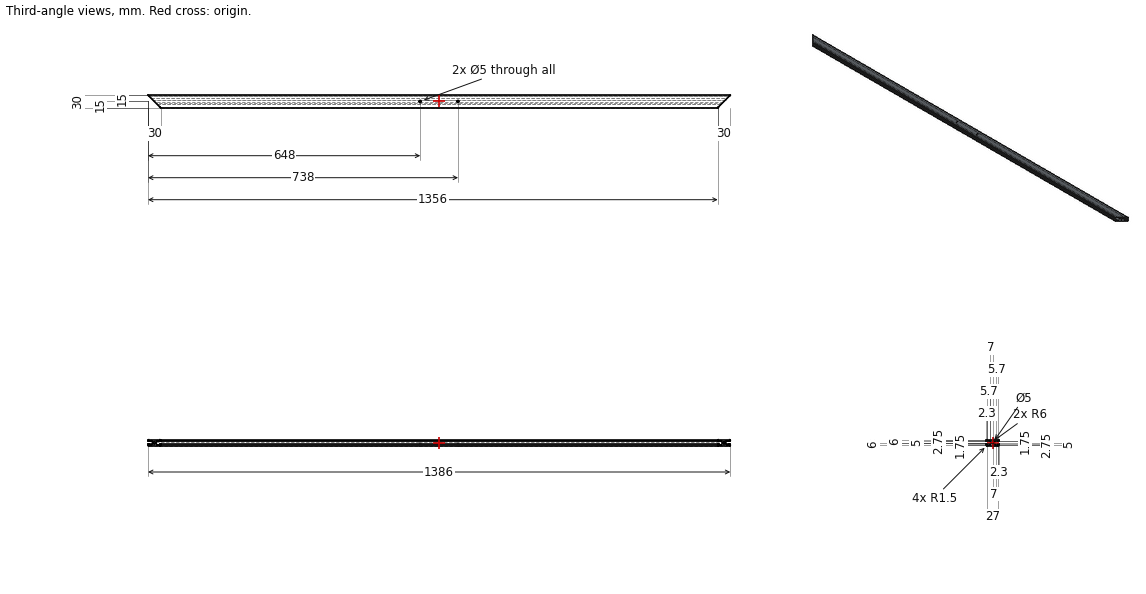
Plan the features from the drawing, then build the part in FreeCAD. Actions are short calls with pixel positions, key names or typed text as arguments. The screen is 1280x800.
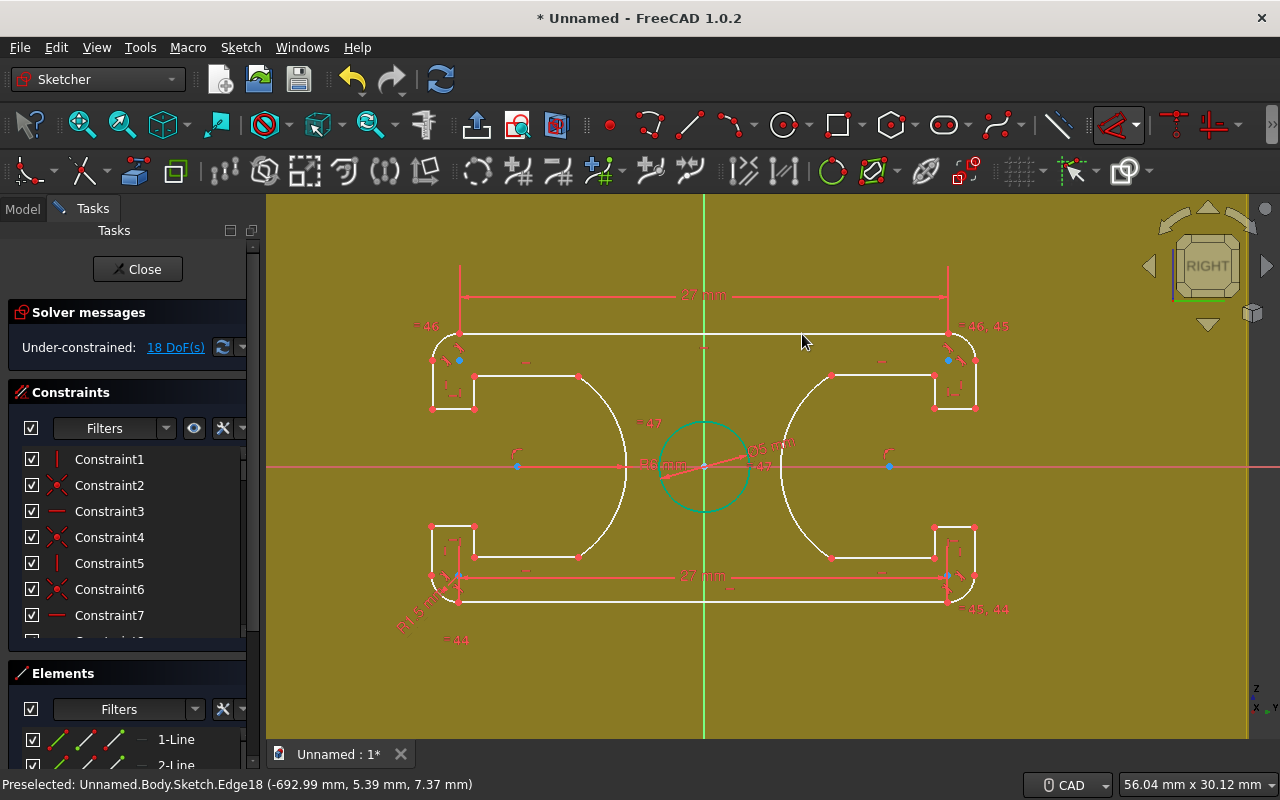
click(433, 361)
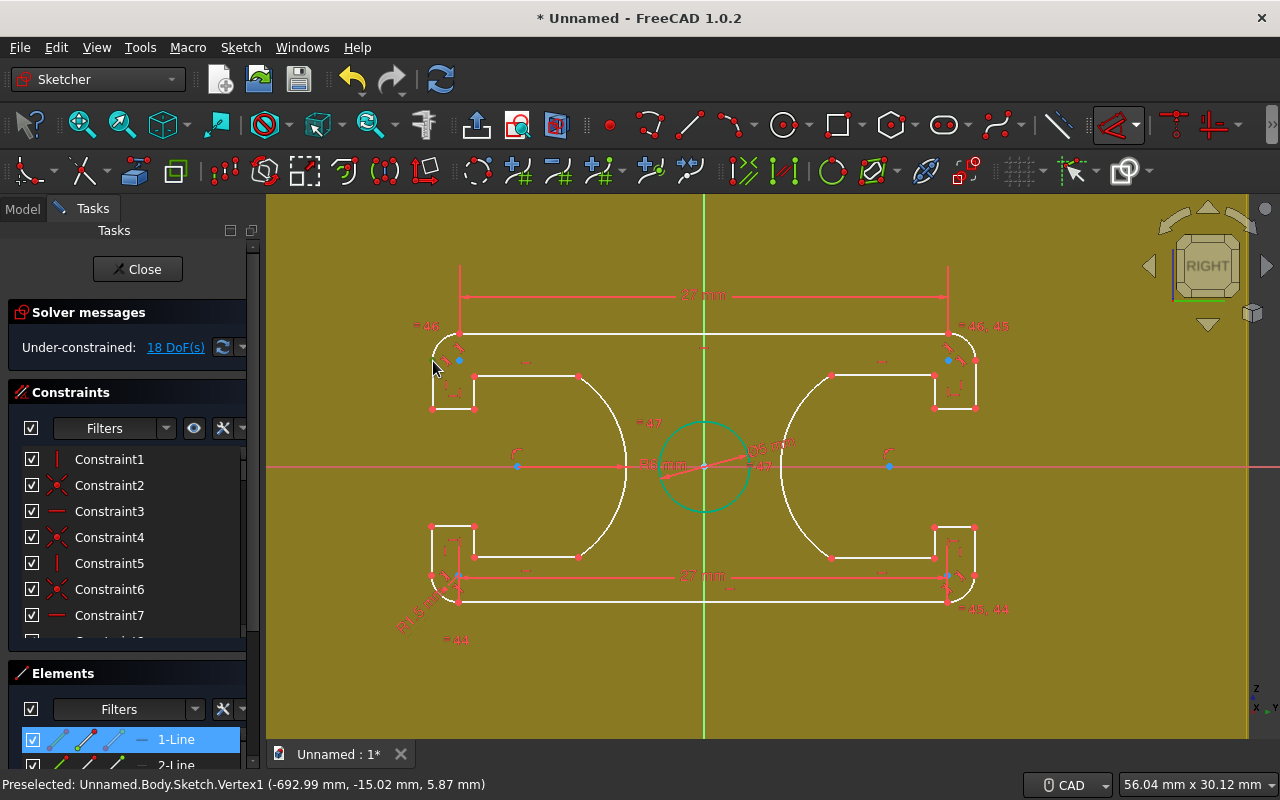
click(1138, 126)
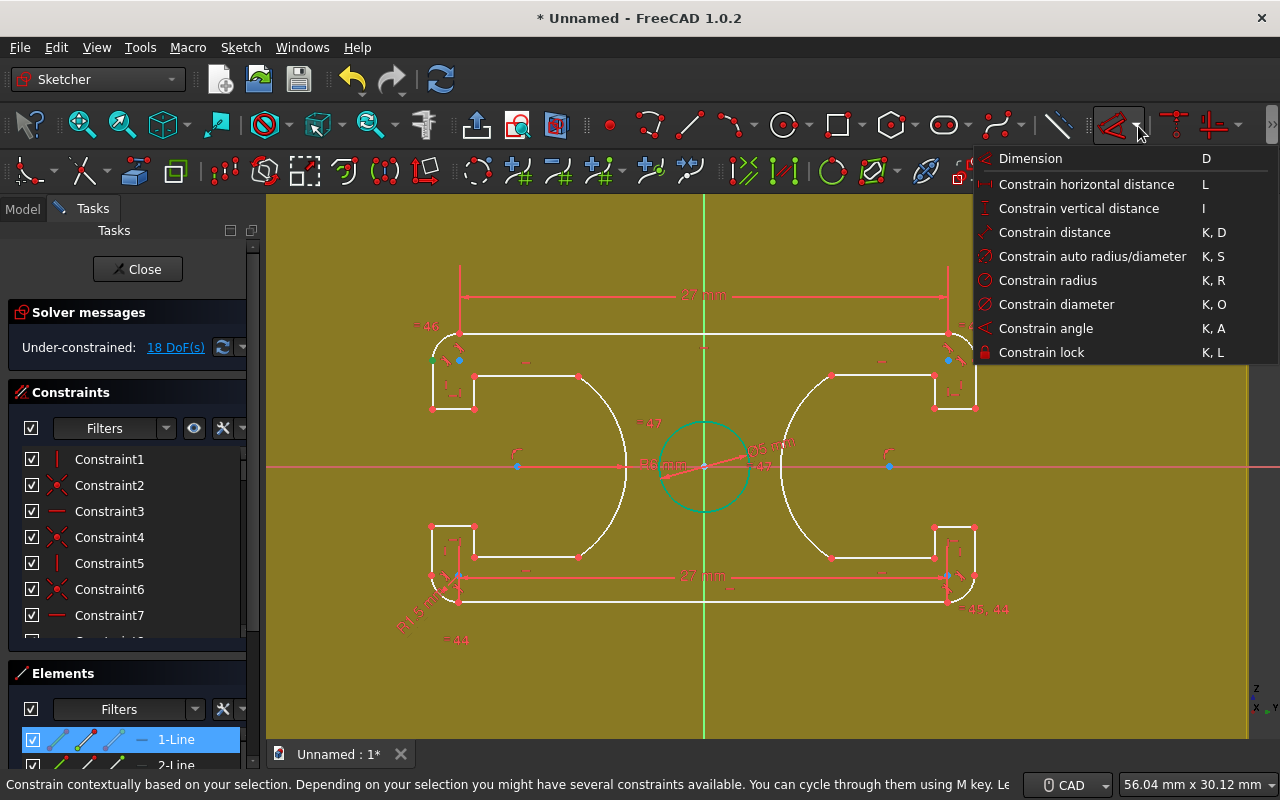
click(1126, 208)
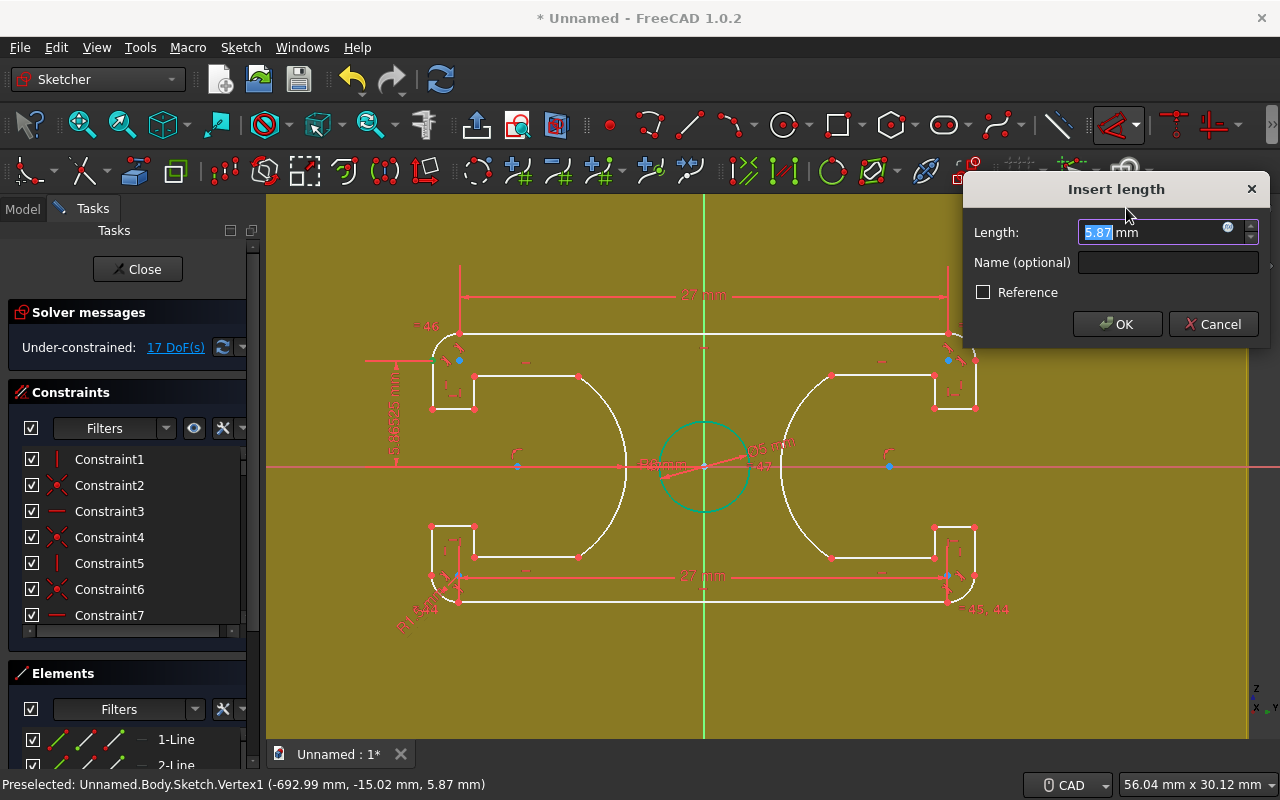
text(6)
key(Return)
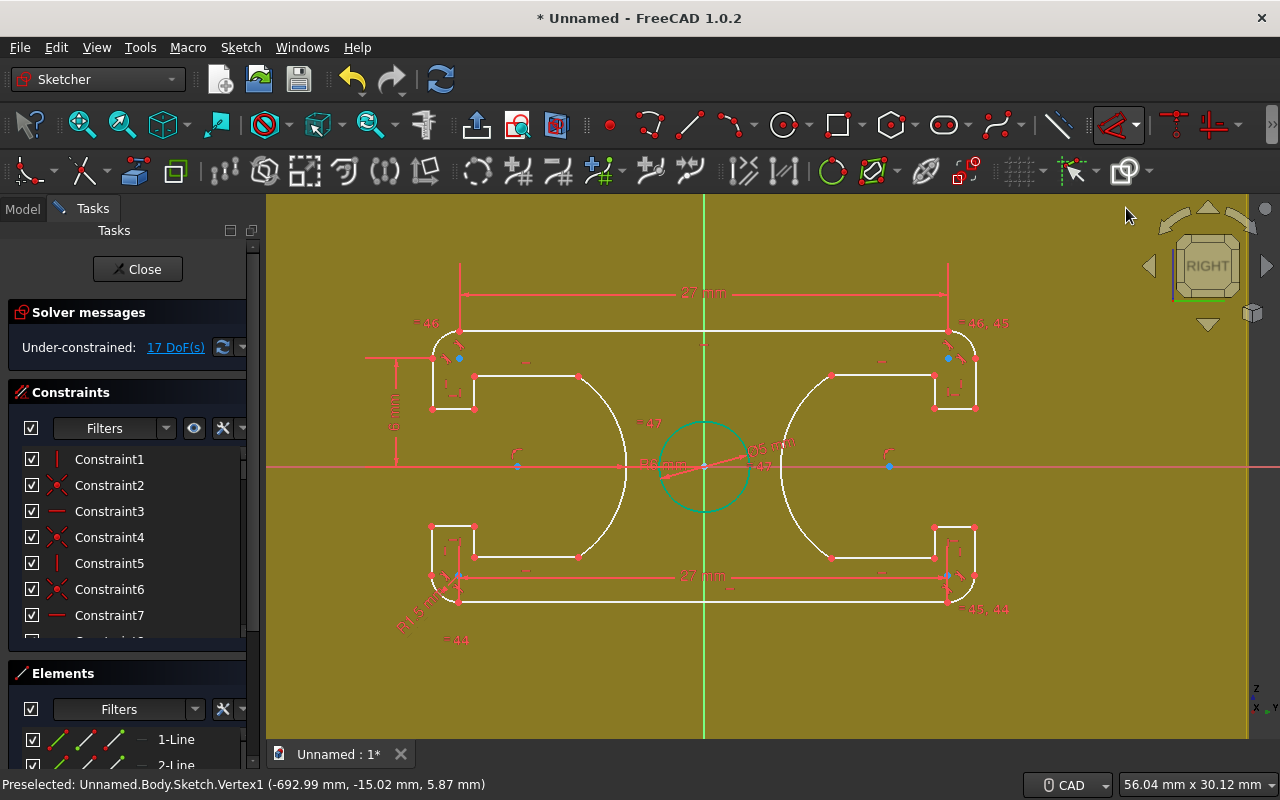
click(474, 376)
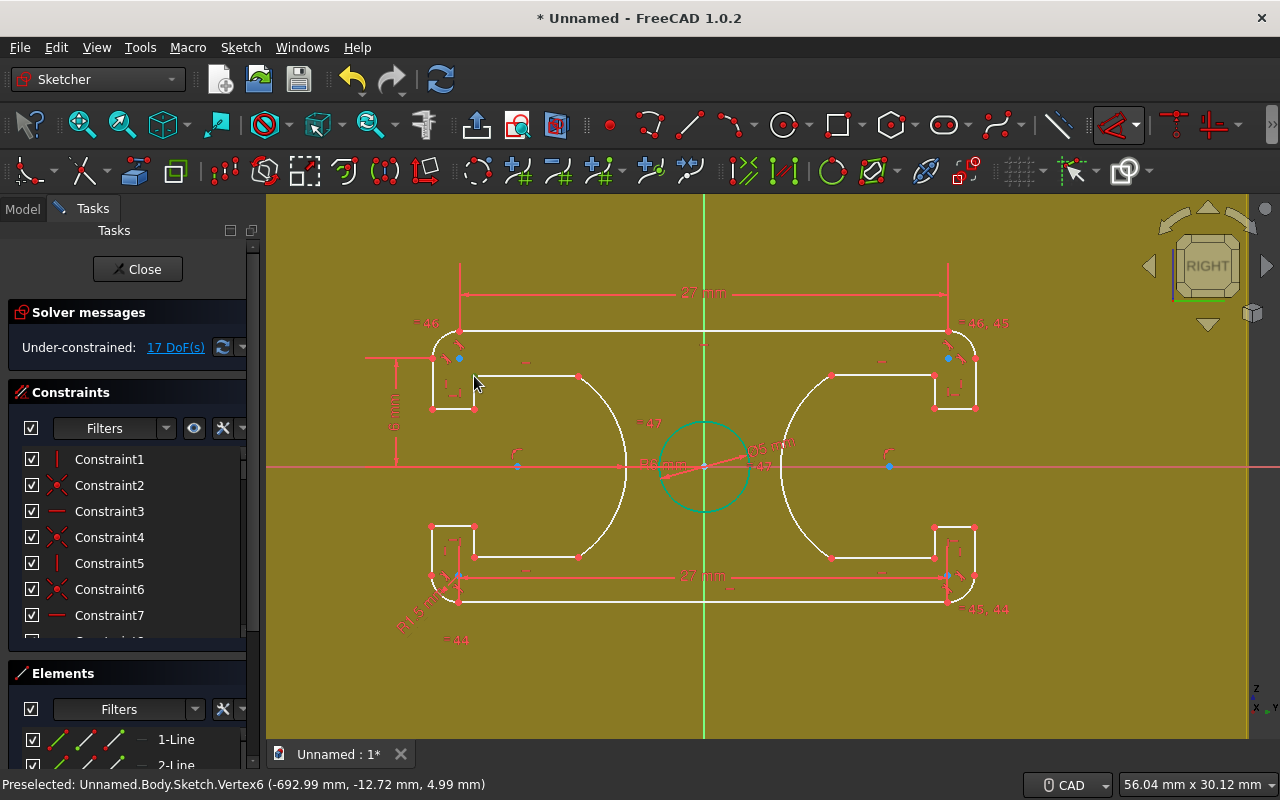
key(i)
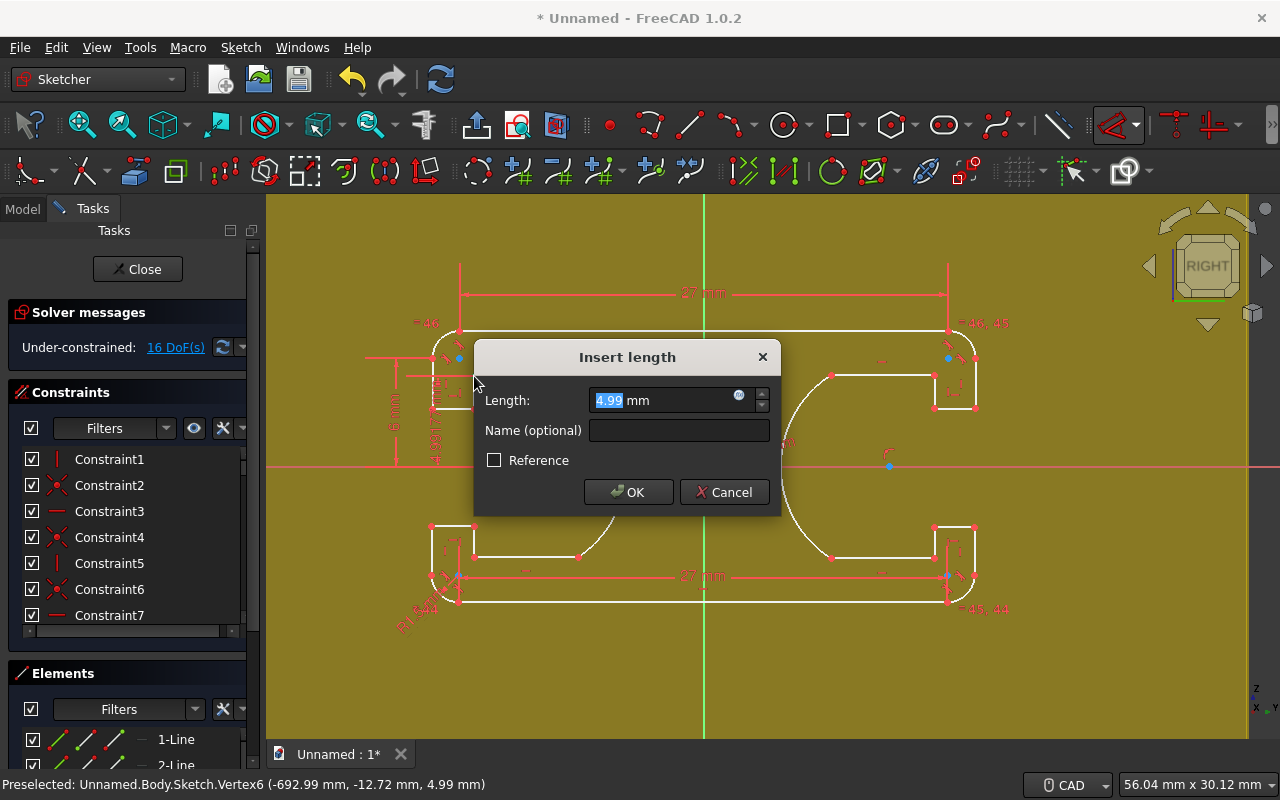
text(5)
key(Return)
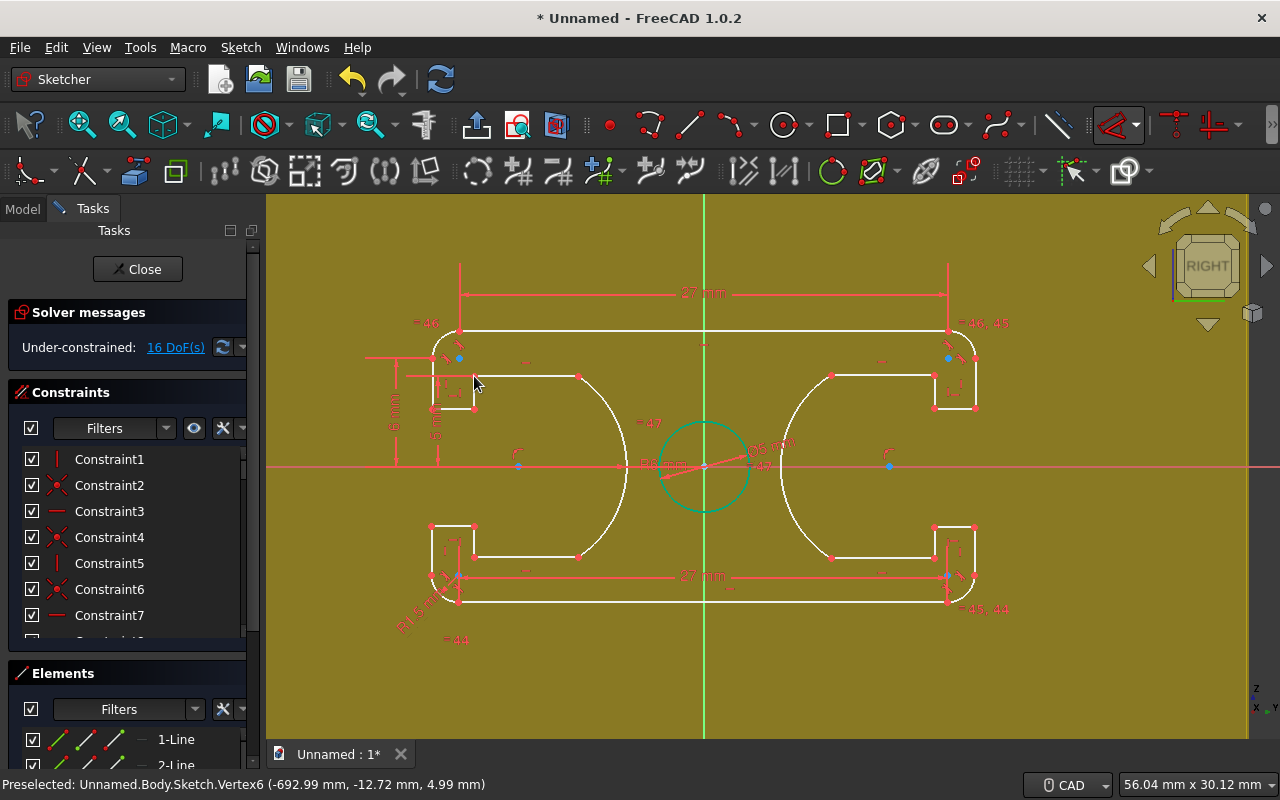
click(578, 376)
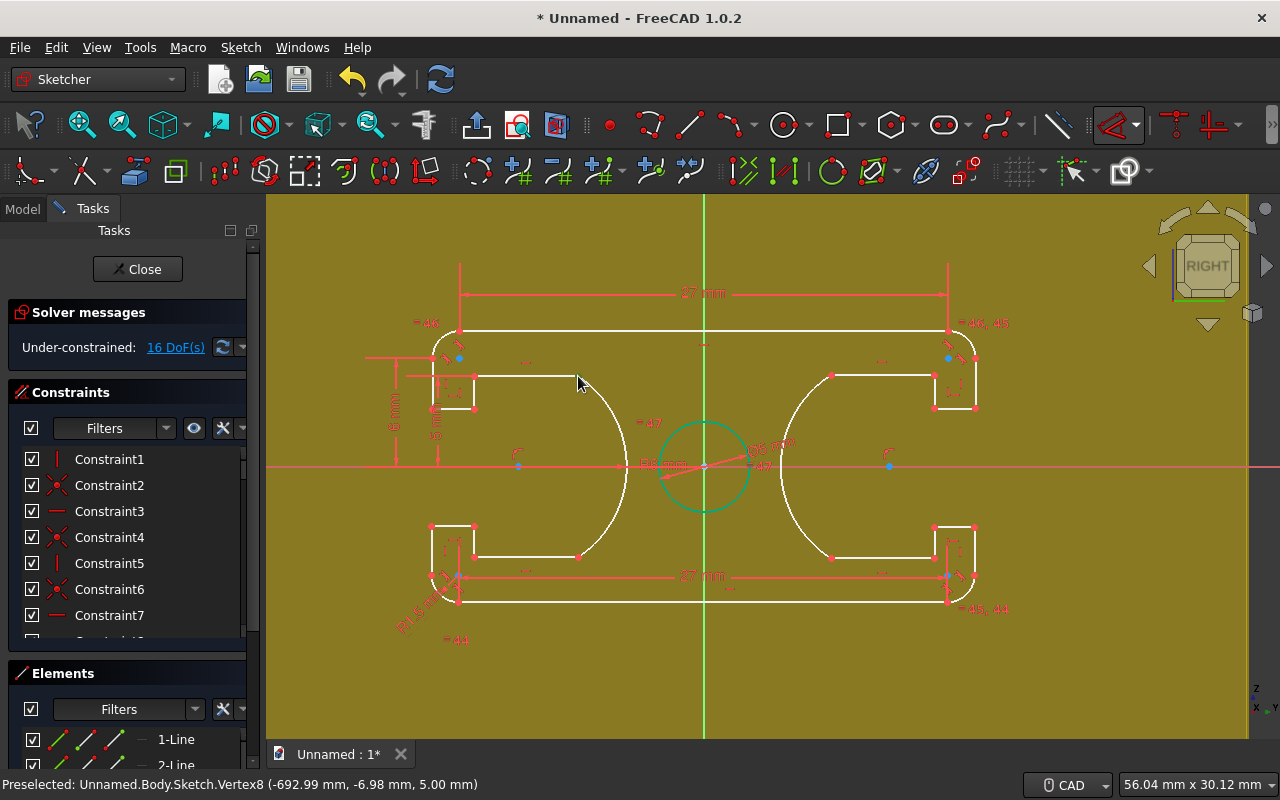
click(1138, 126)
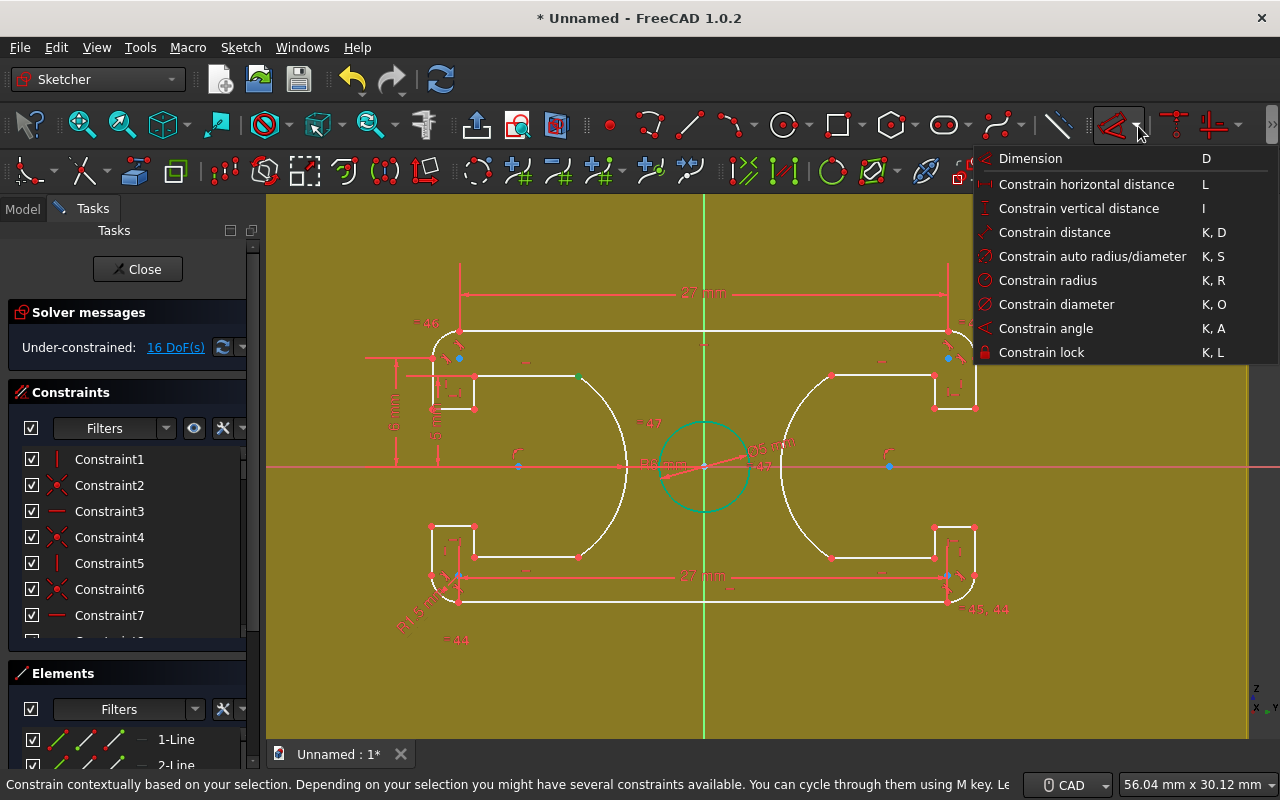
click(1126, 184)